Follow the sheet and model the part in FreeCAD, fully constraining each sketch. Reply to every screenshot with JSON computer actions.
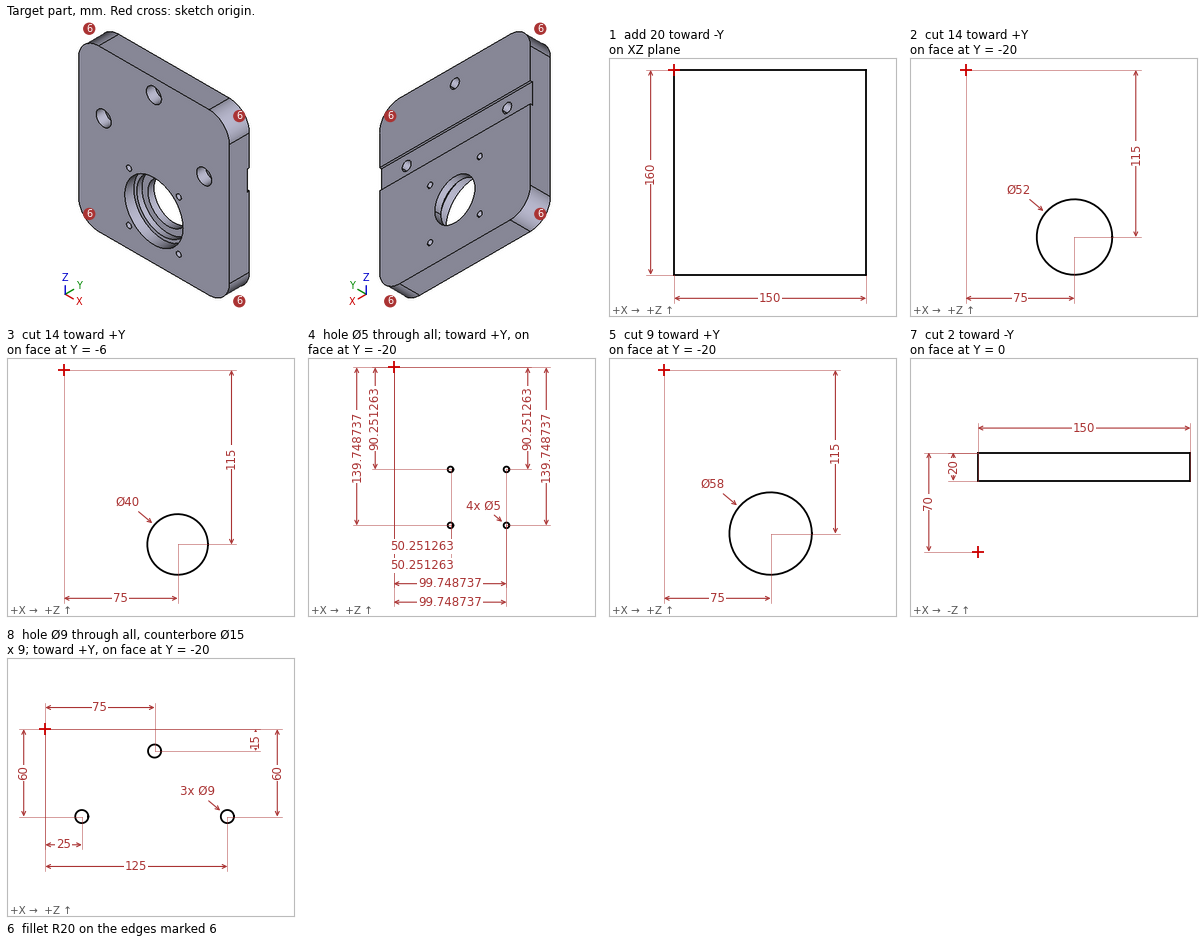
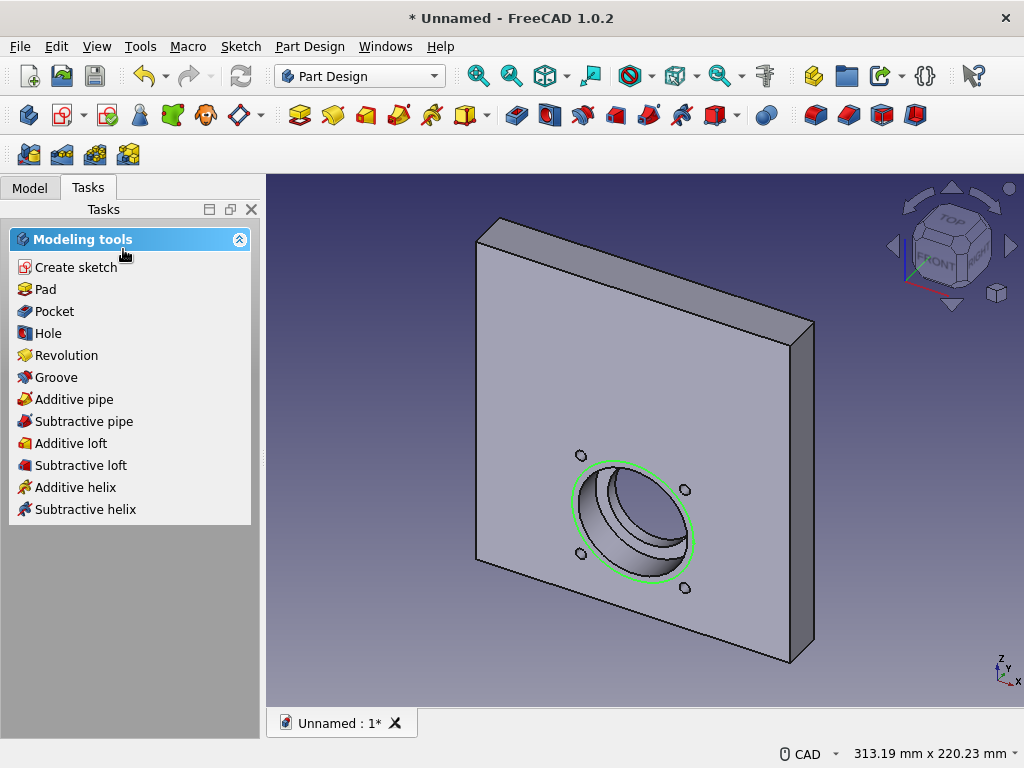
{"action": "left_click", "coordinate": [517, 116]}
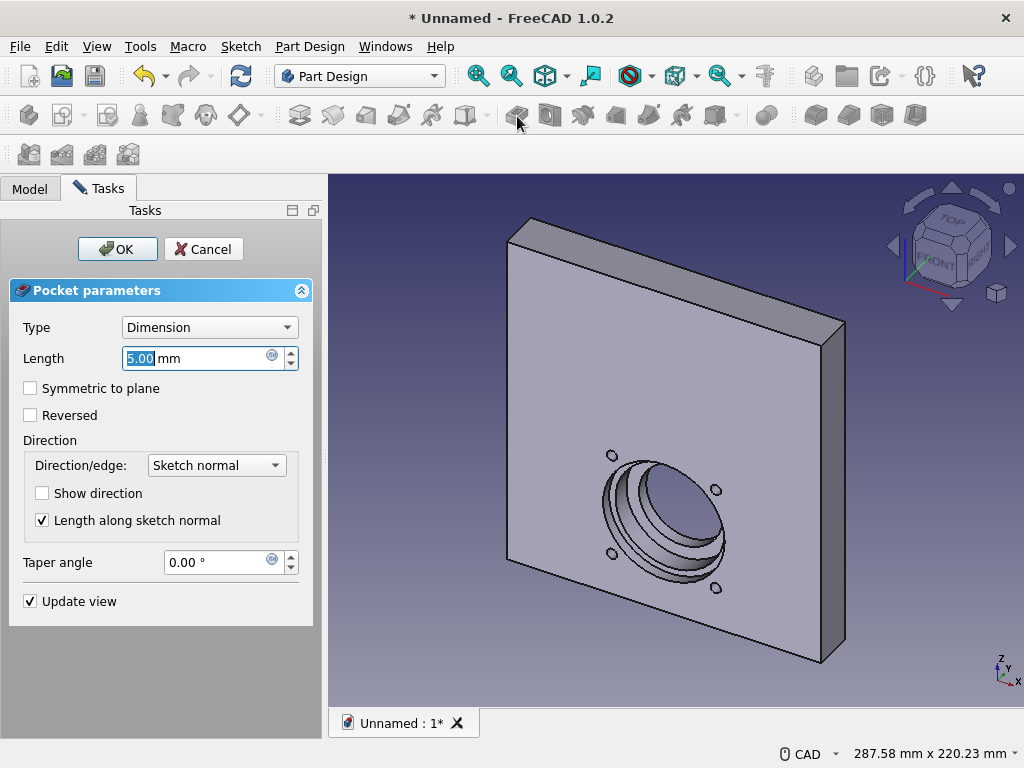
{"action": "type", "text": "9"}
{"action": "key", "text": "Tab"}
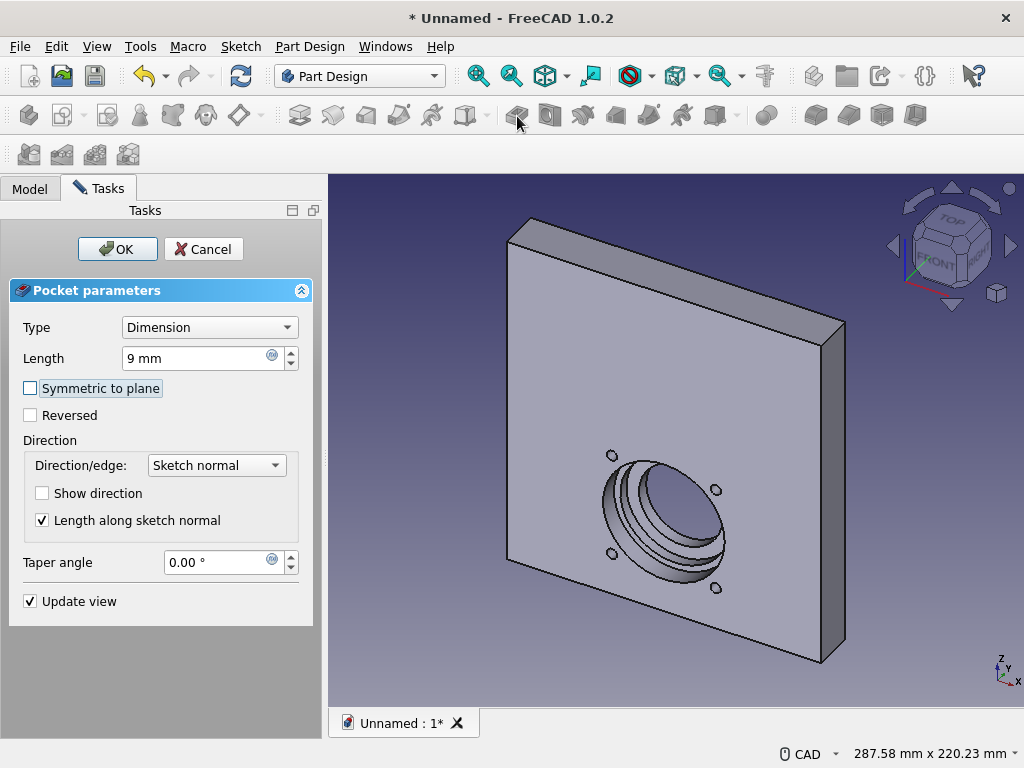
{"action": "left_click", "coordinate": [118, 249]}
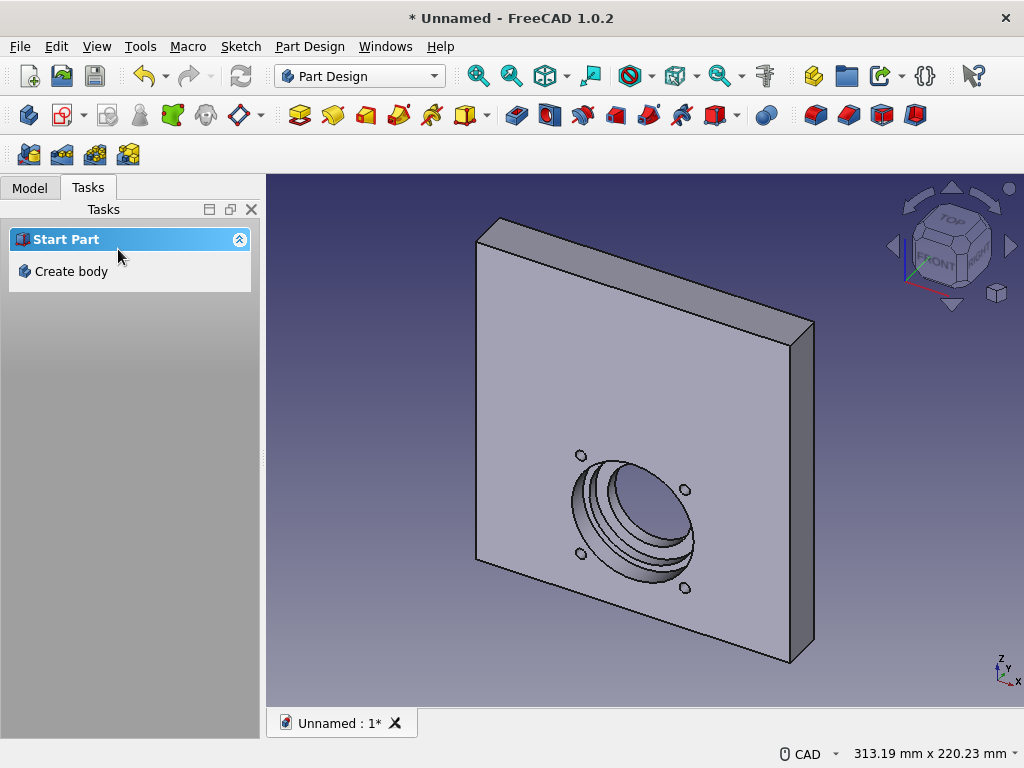
{"action": "left_click", "coordinate": [802, 333]}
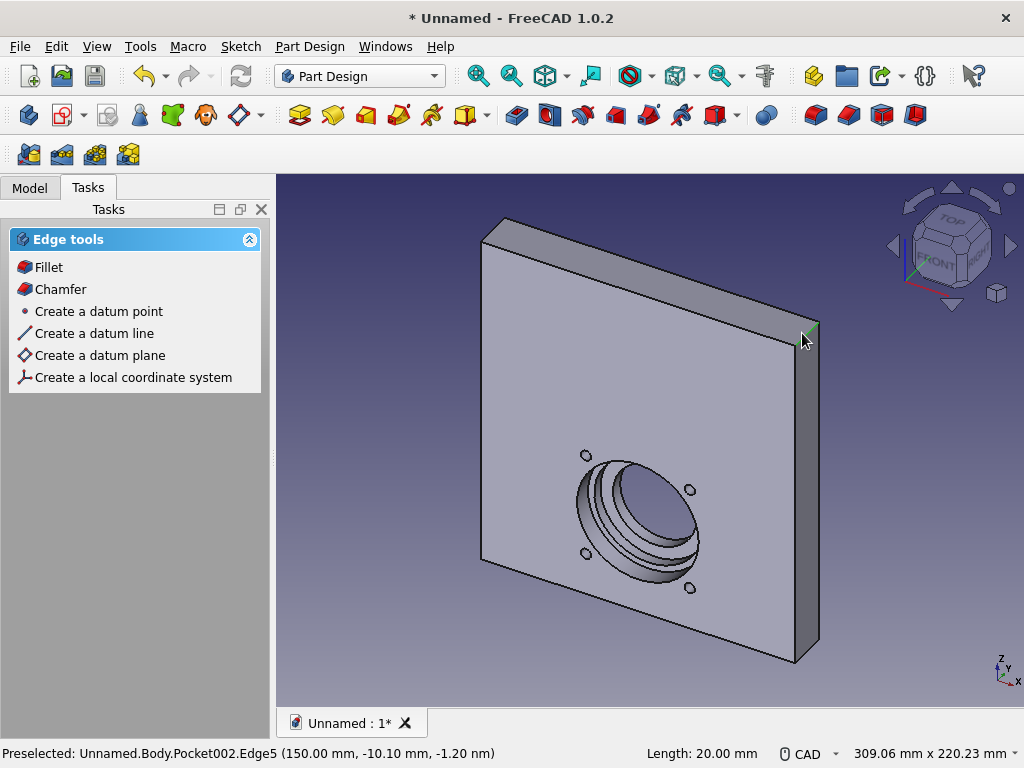
{"action": "key", "text": "0"}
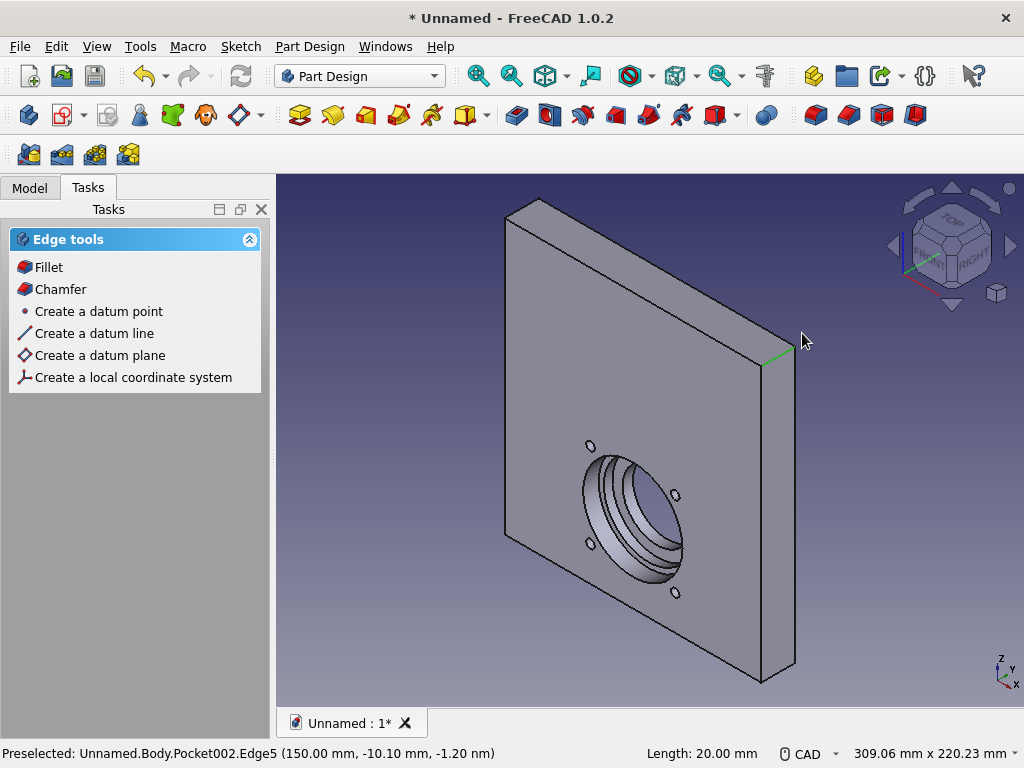
{"action": "key", "text": "2"}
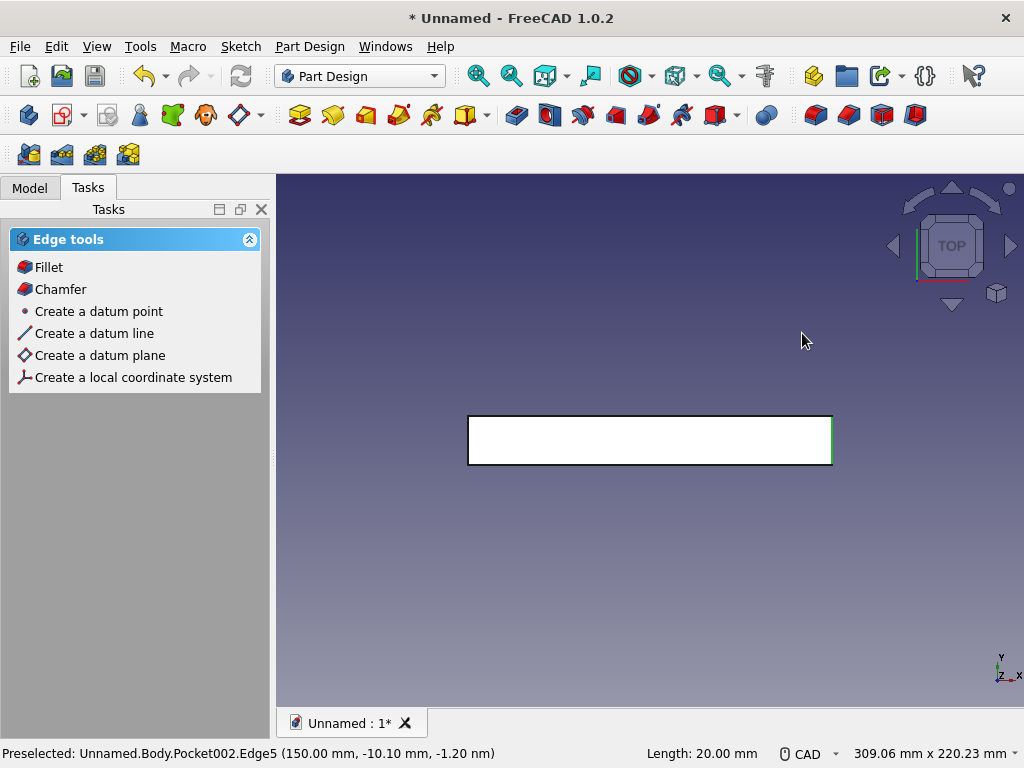
{"action": "left_click", "coordinate": [468, 440], "text": "ctrl"}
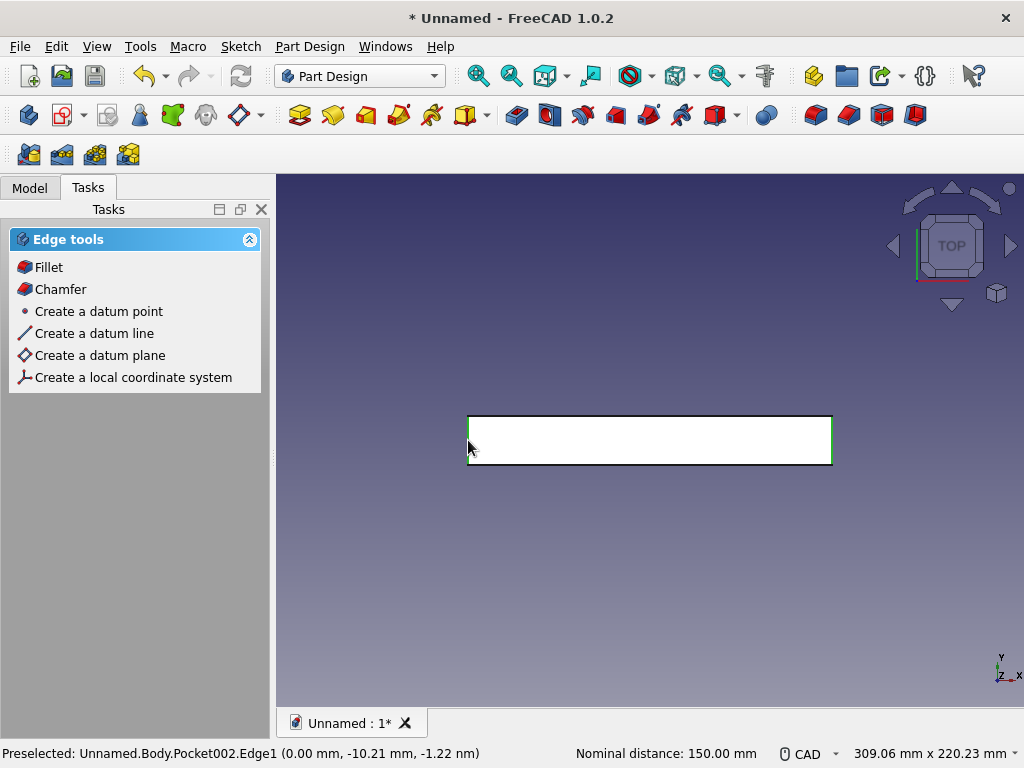
{"action": "key", "text": "1"}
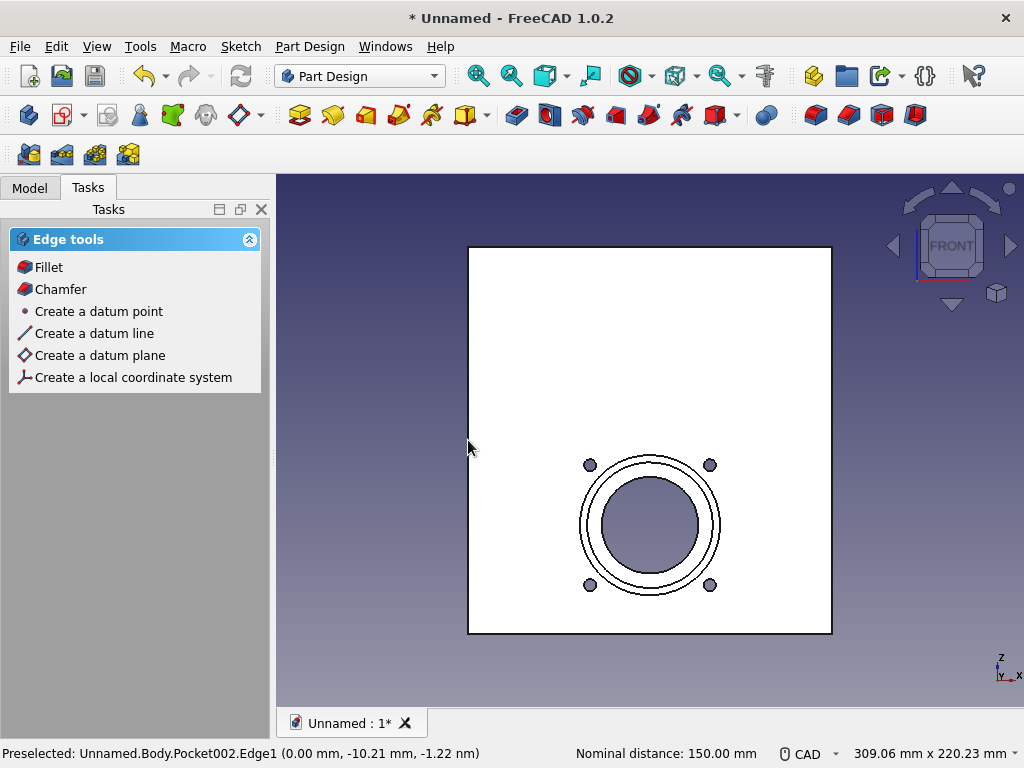
{"action": "key", "text": "3"}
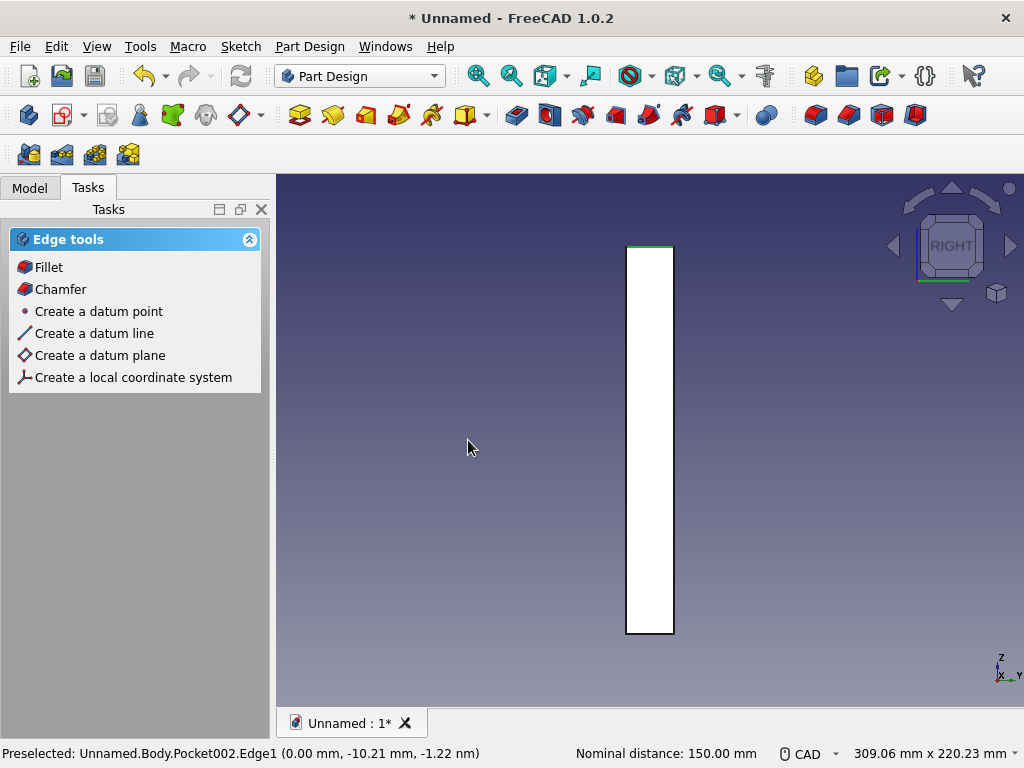
{"action": "left_click", "coordinate": [650, 633], "text": "ctrl"}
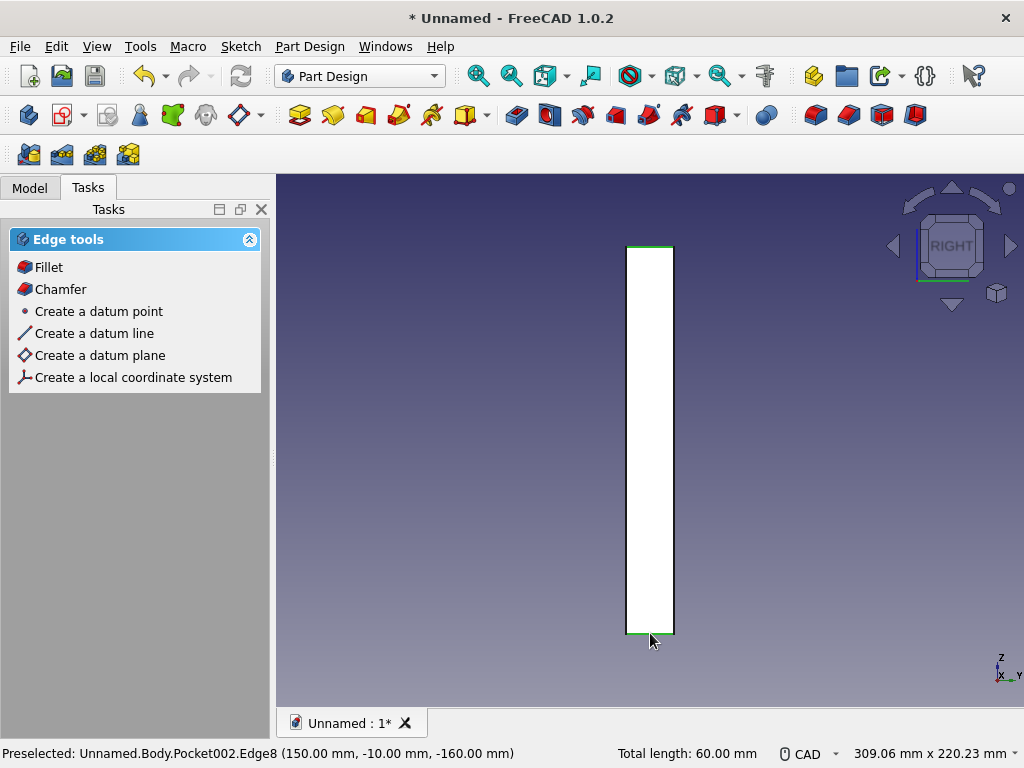
{"action": "key", "text": "5"}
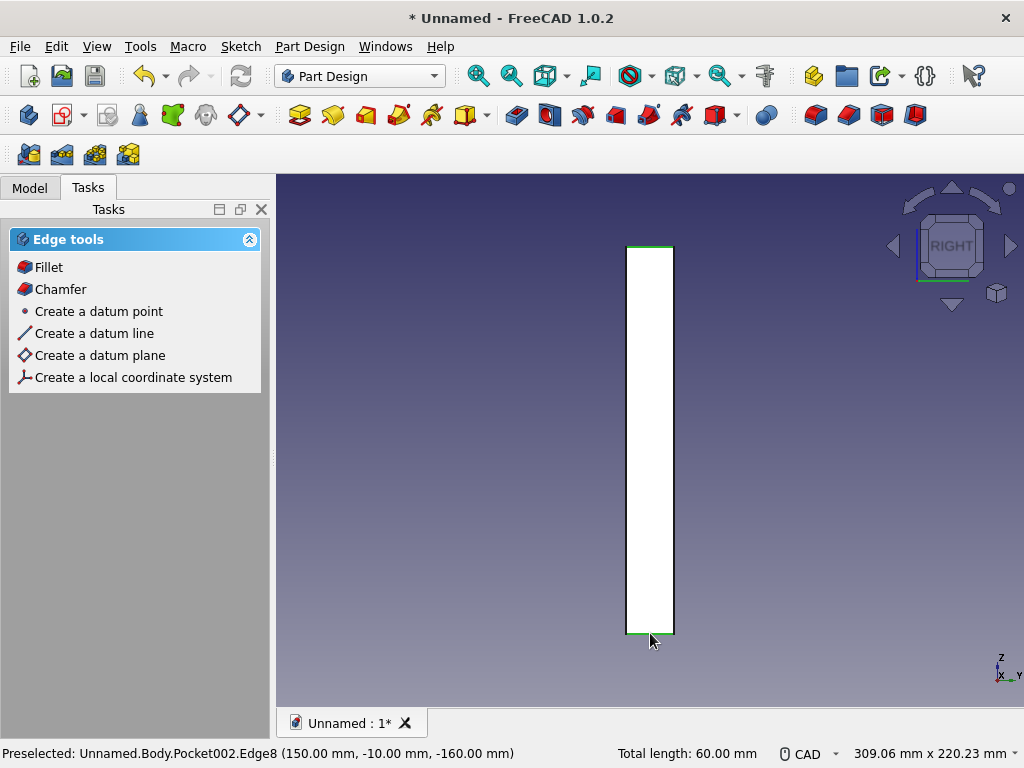
{"action": "left_click", "coordinate": [468, 439], "text": "ctrl"}